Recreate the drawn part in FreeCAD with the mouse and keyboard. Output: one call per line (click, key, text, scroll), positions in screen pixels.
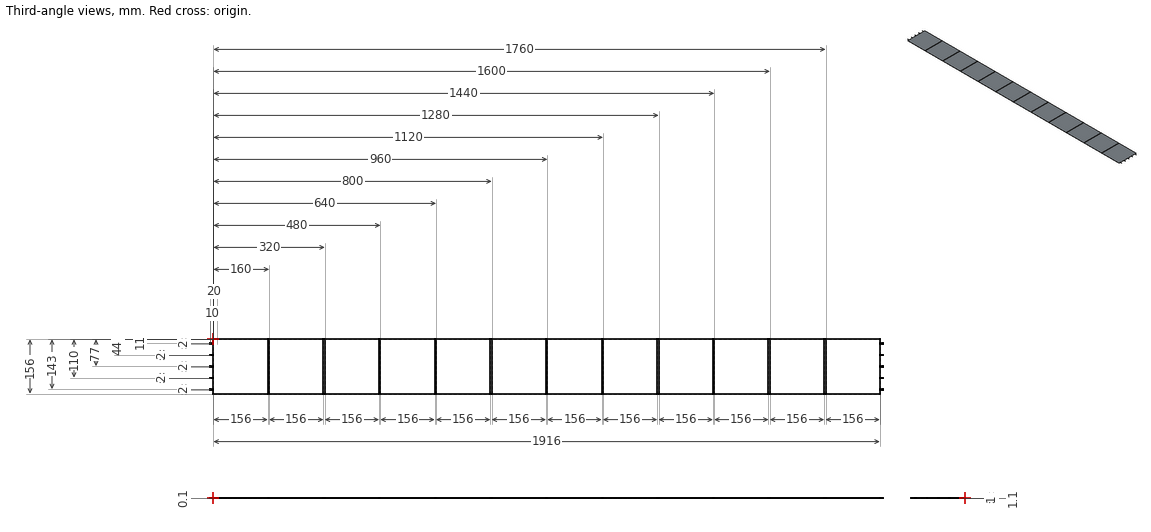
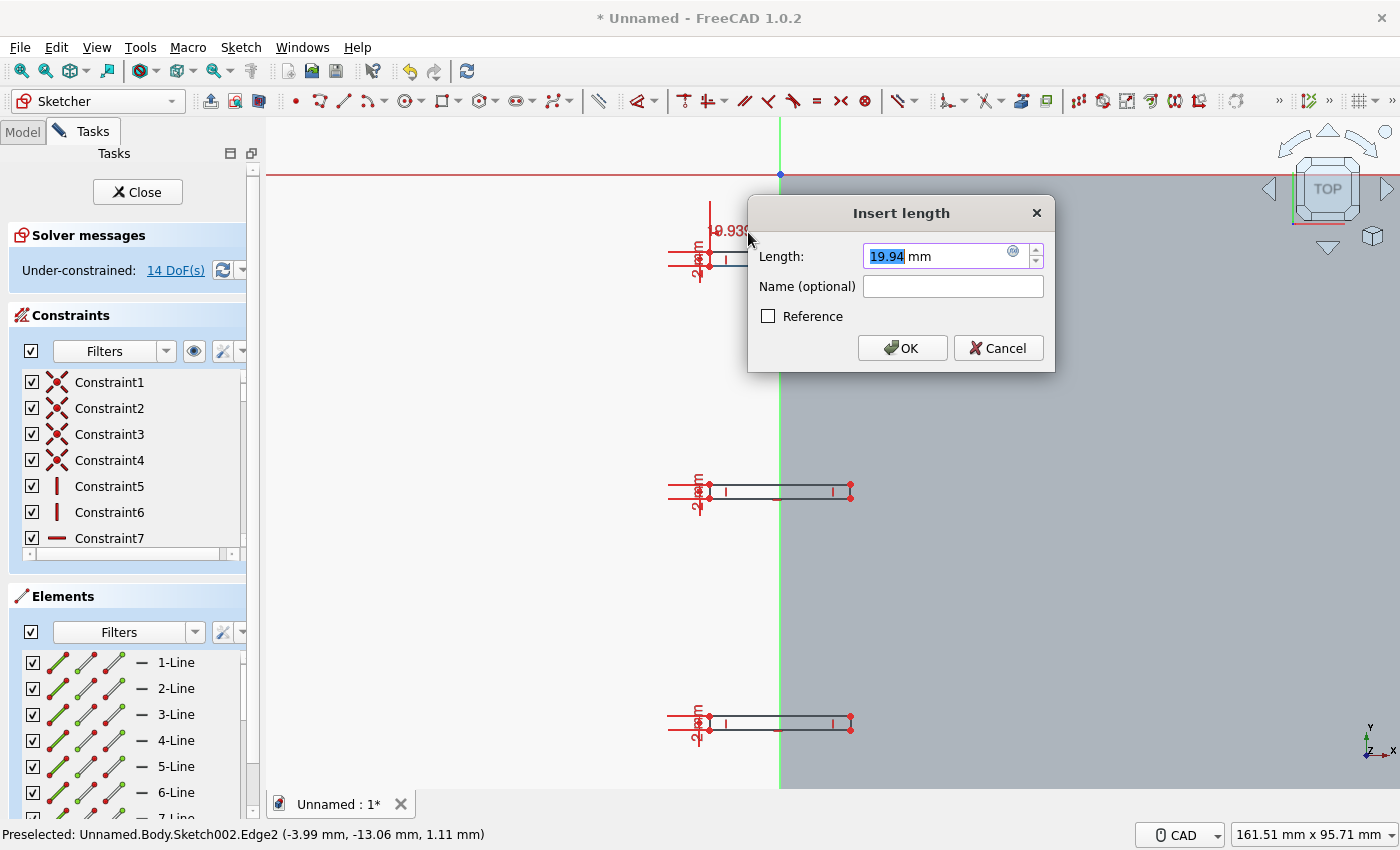
text(20)
key(Return)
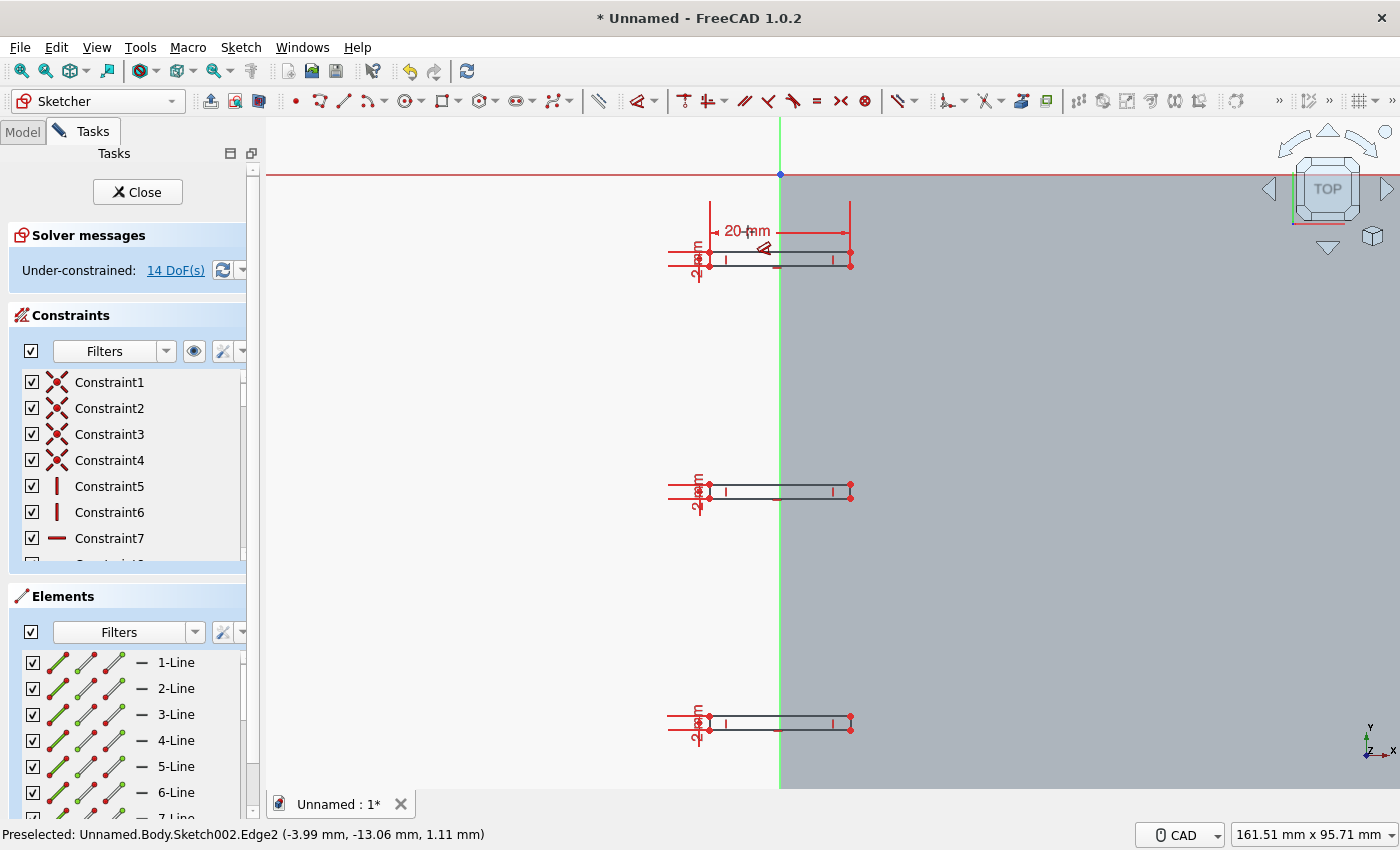
click(752, 499)
click(748, 465)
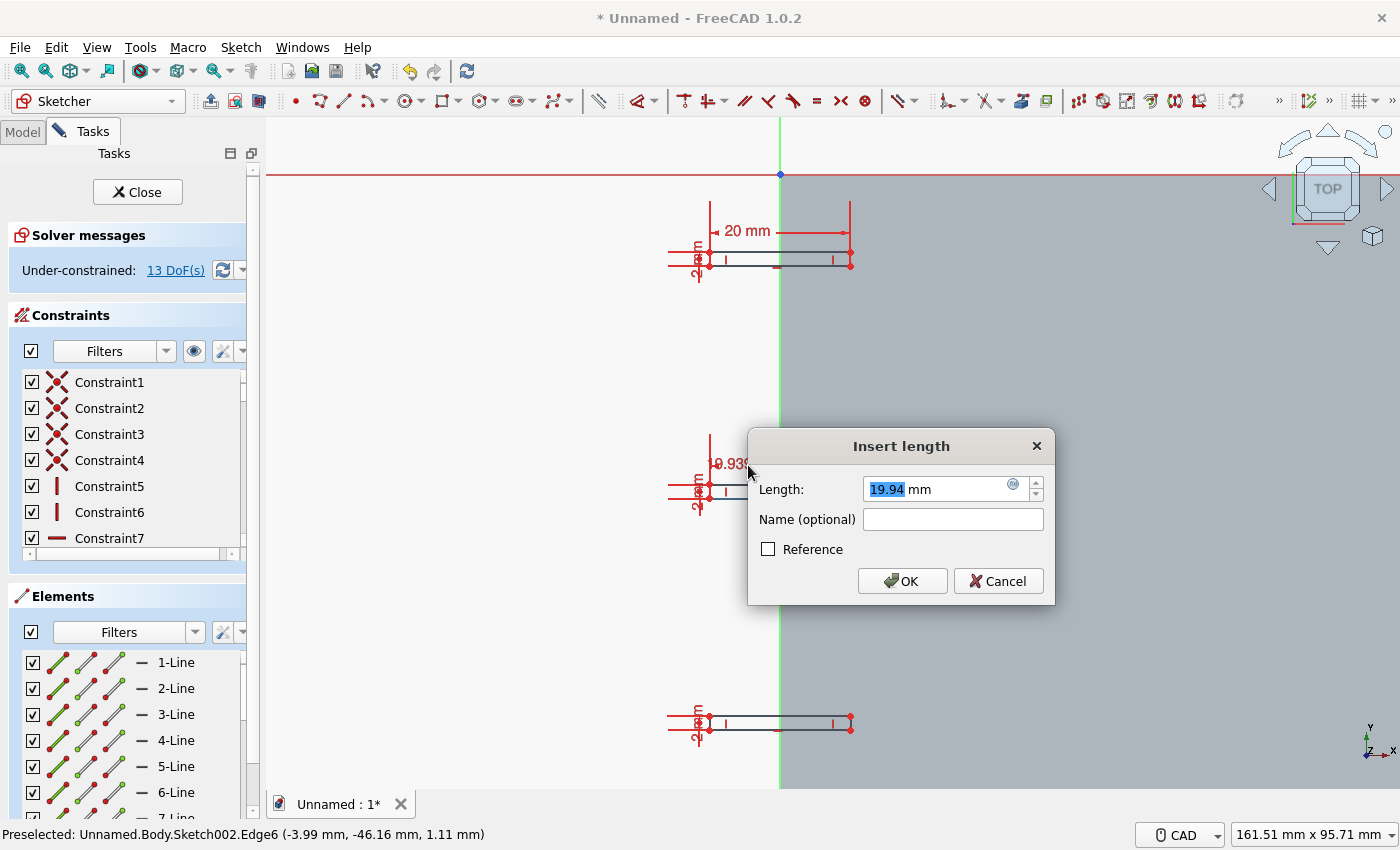
text(20)
key(Return)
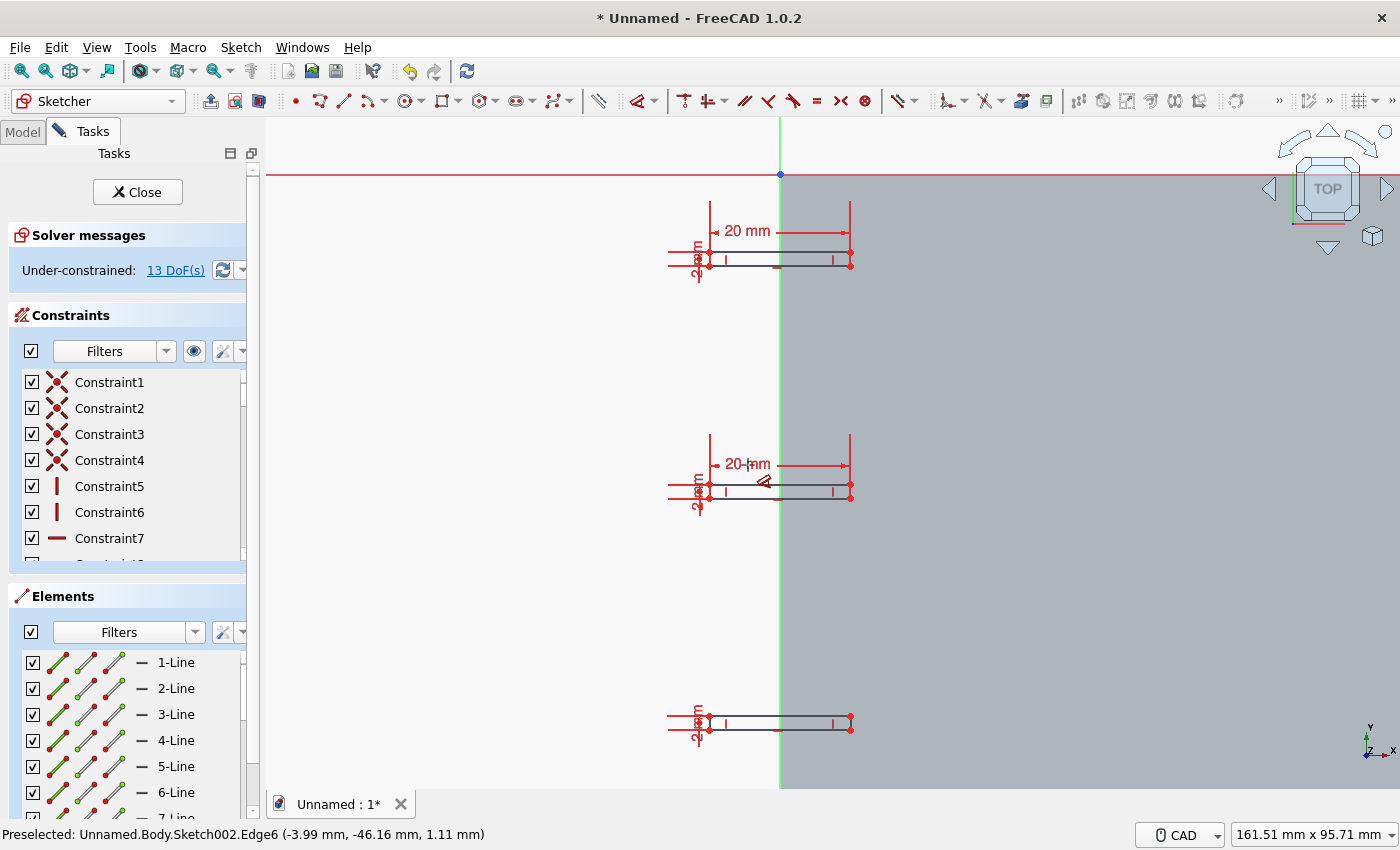
click(752, 730)
click(748, 696)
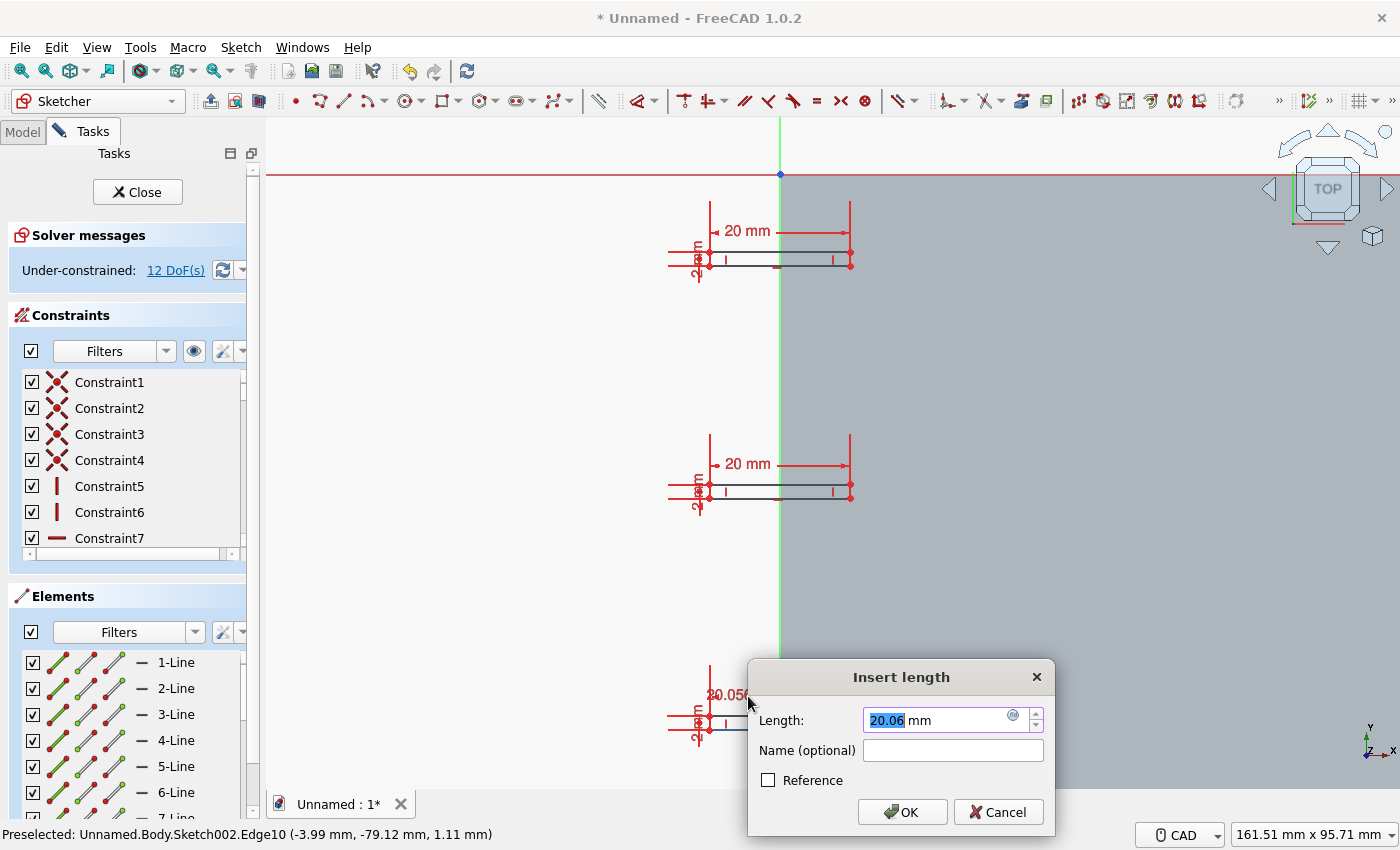
text(20)
key(Return)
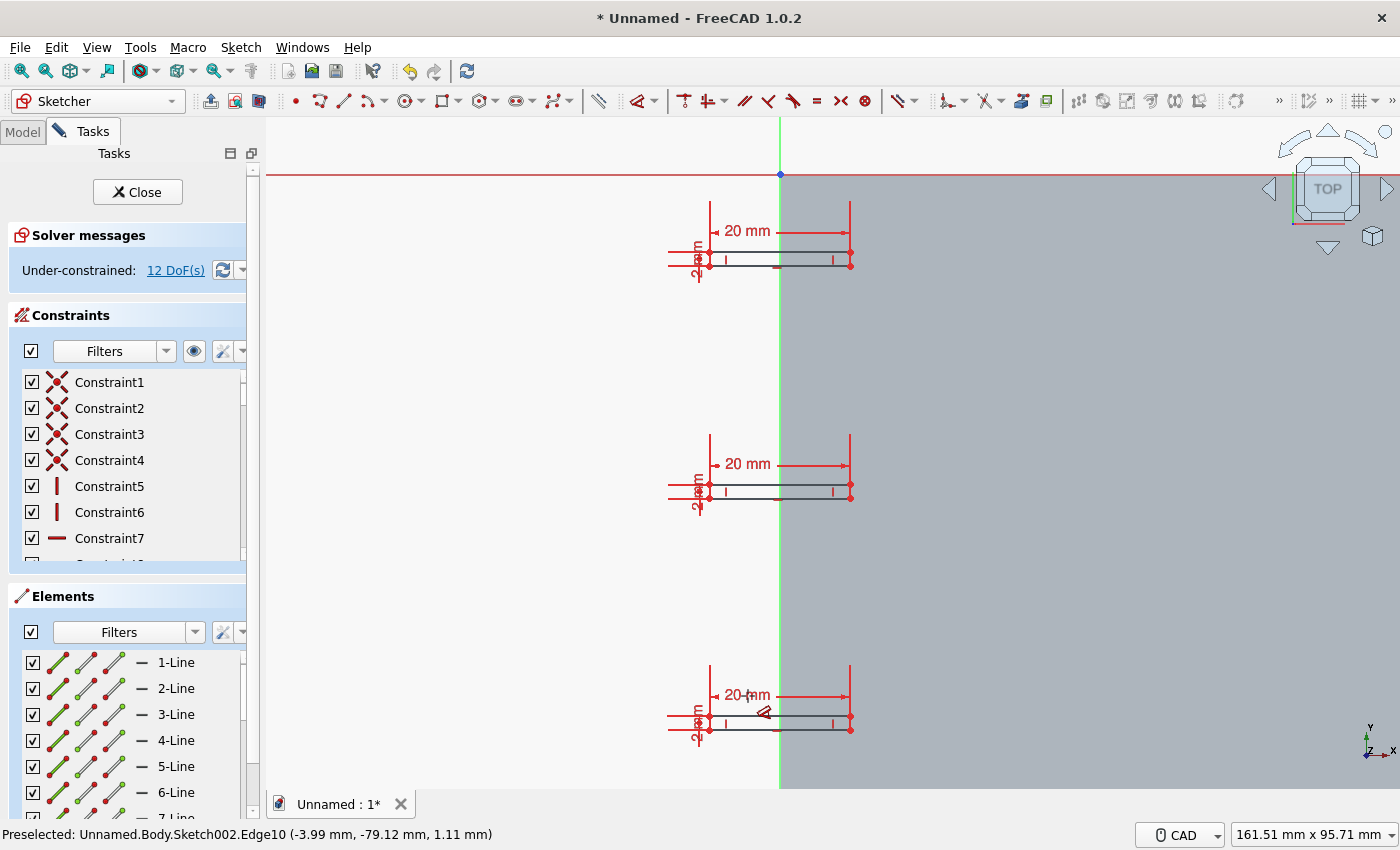
scroll(752, 265, down, 4)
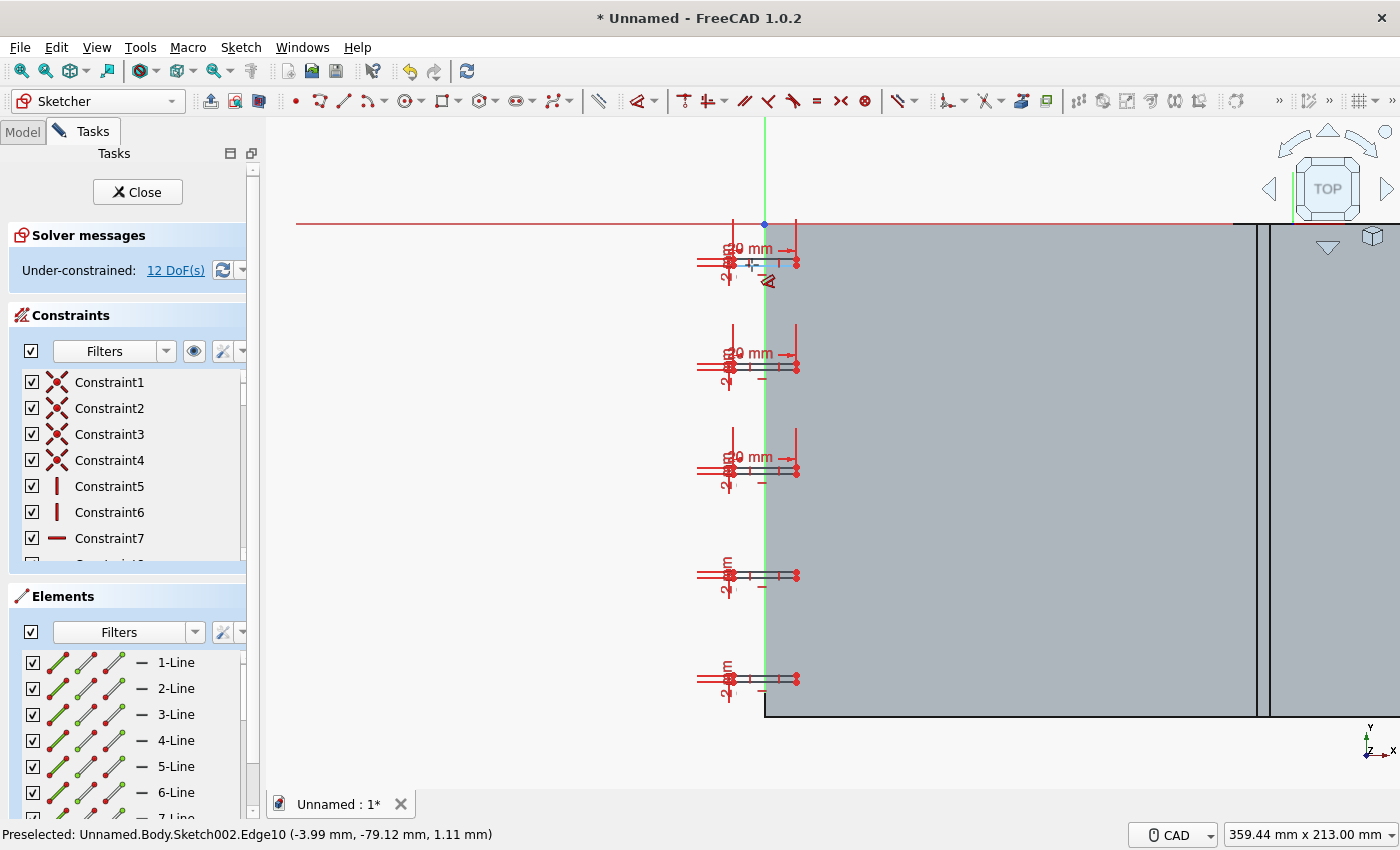
scroll(752, 578, up, 4)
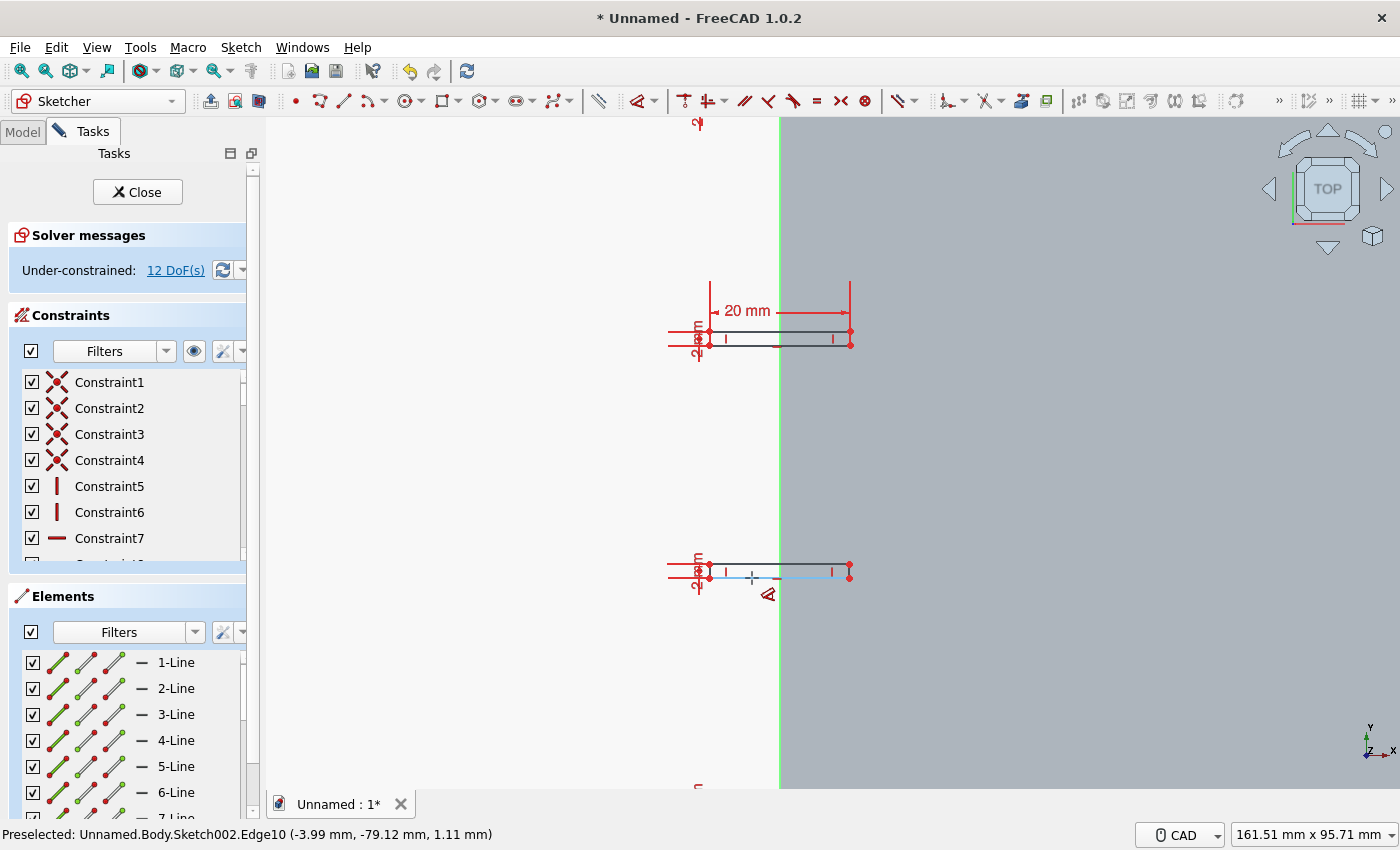
click(752, 578)
click(747, 612)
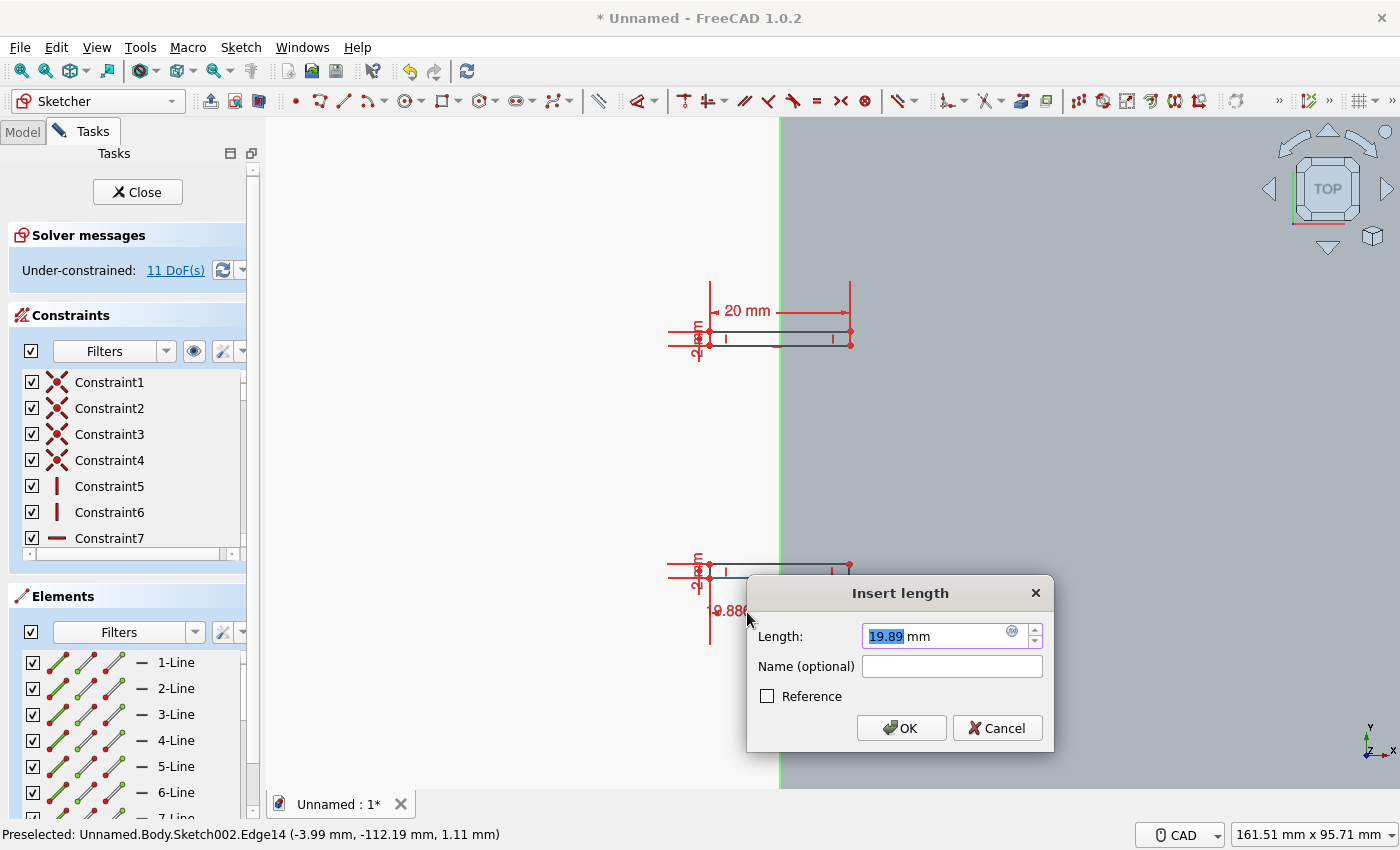
text(20)
key(Return)